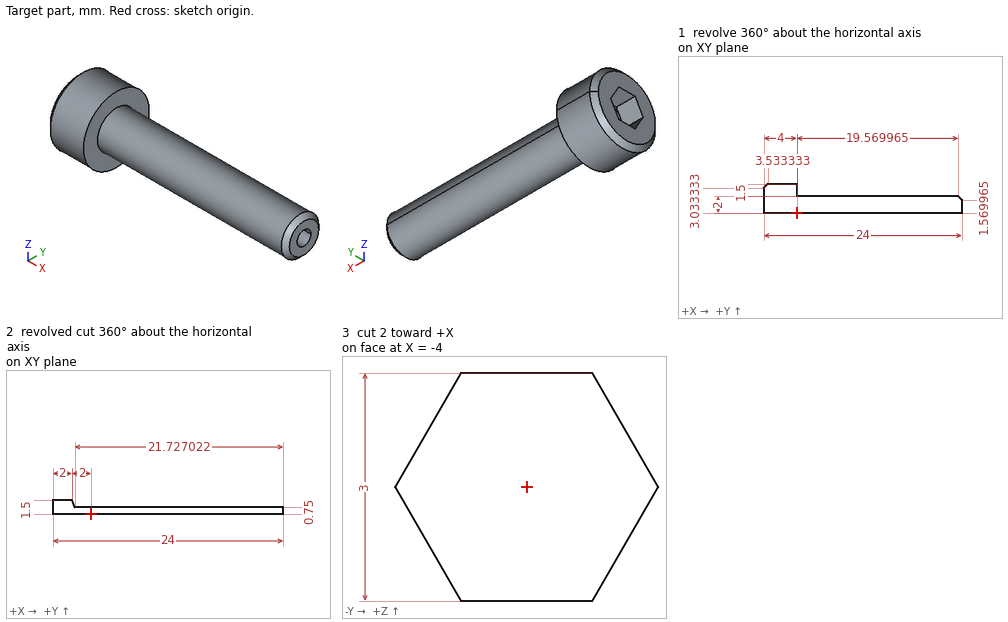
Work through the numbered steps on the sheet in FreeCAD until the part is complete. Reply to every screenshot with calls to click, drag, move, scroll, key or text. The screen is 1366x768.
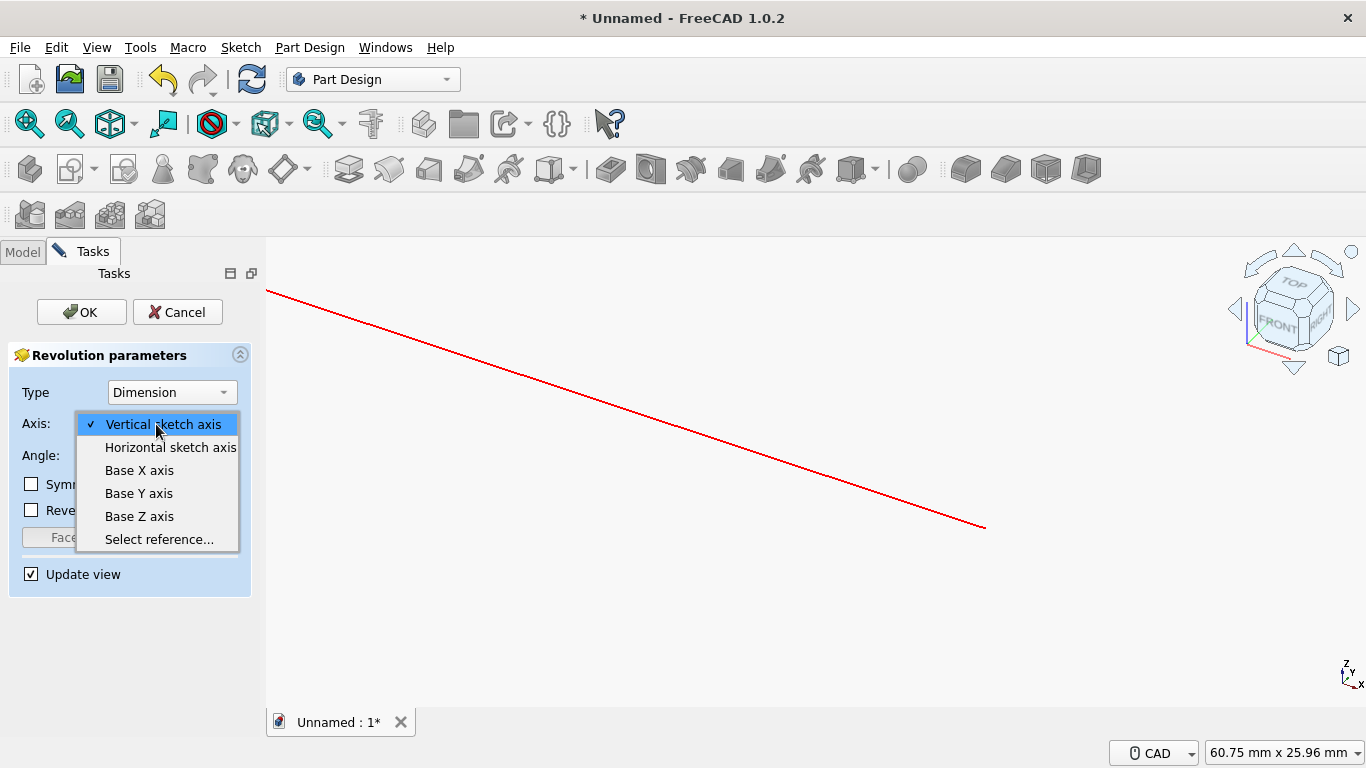
click(156, 448)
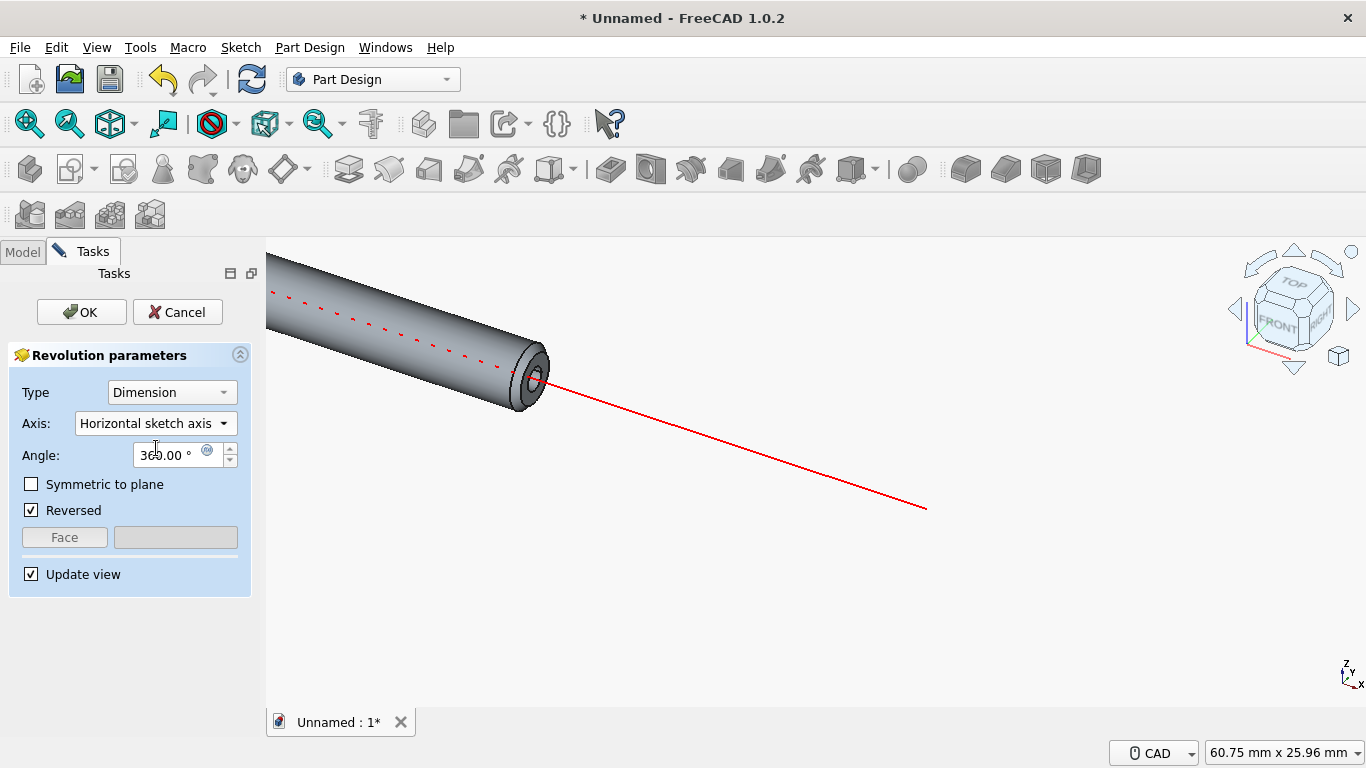
click(82, 312)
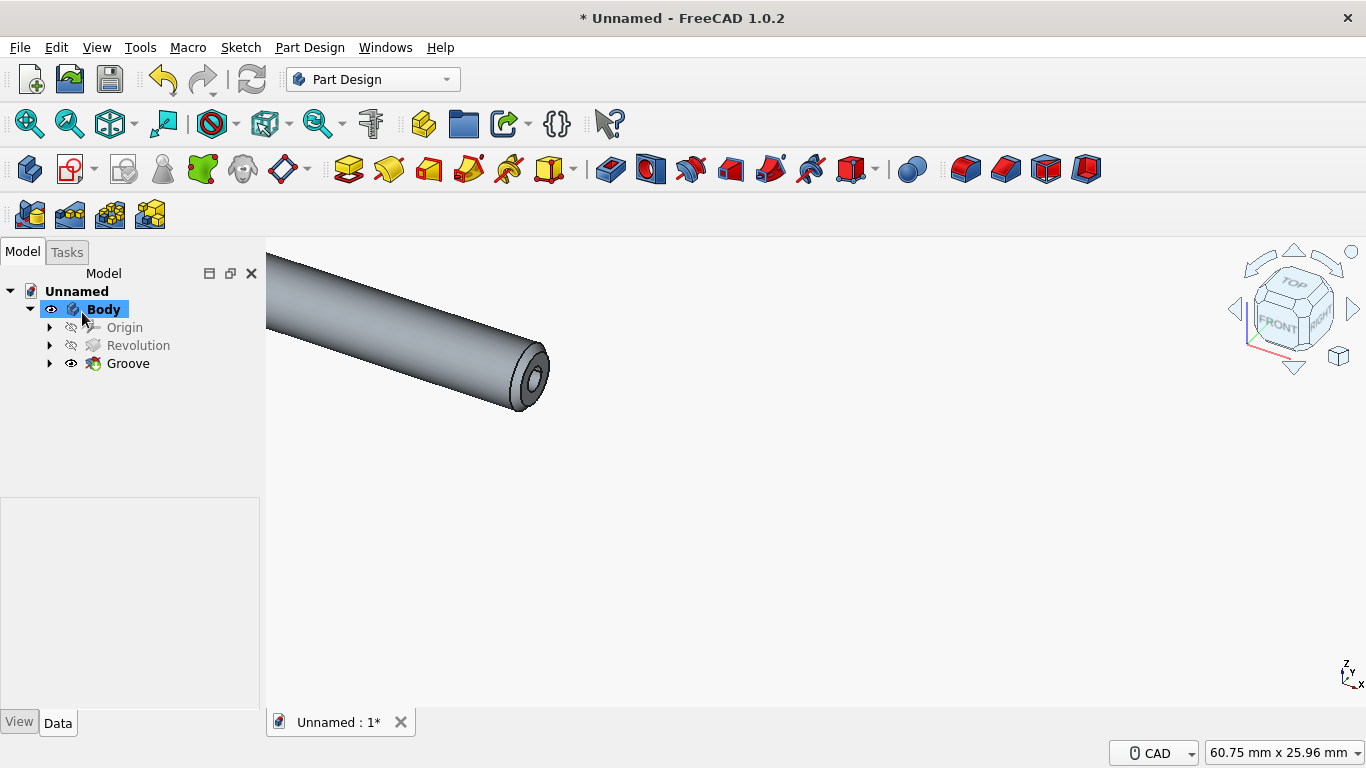
click(30, 124)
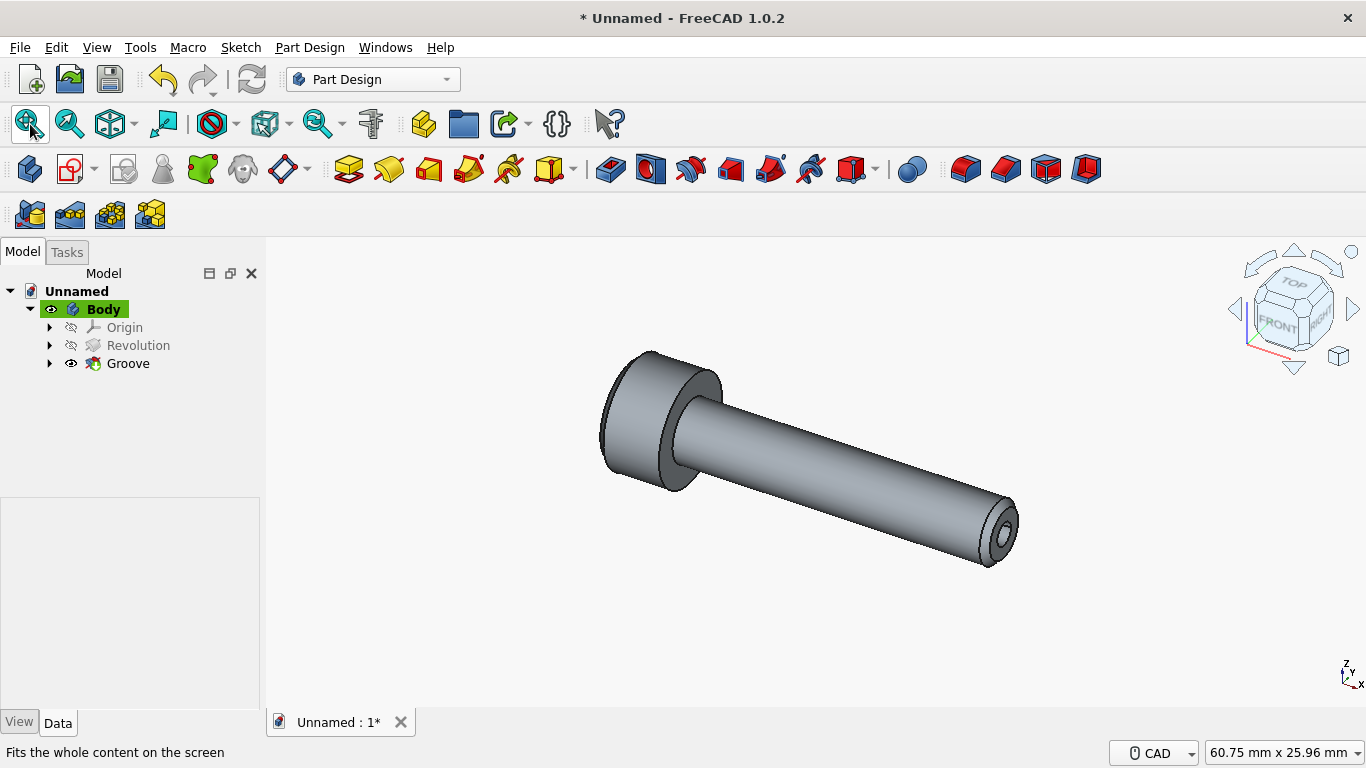
key(6)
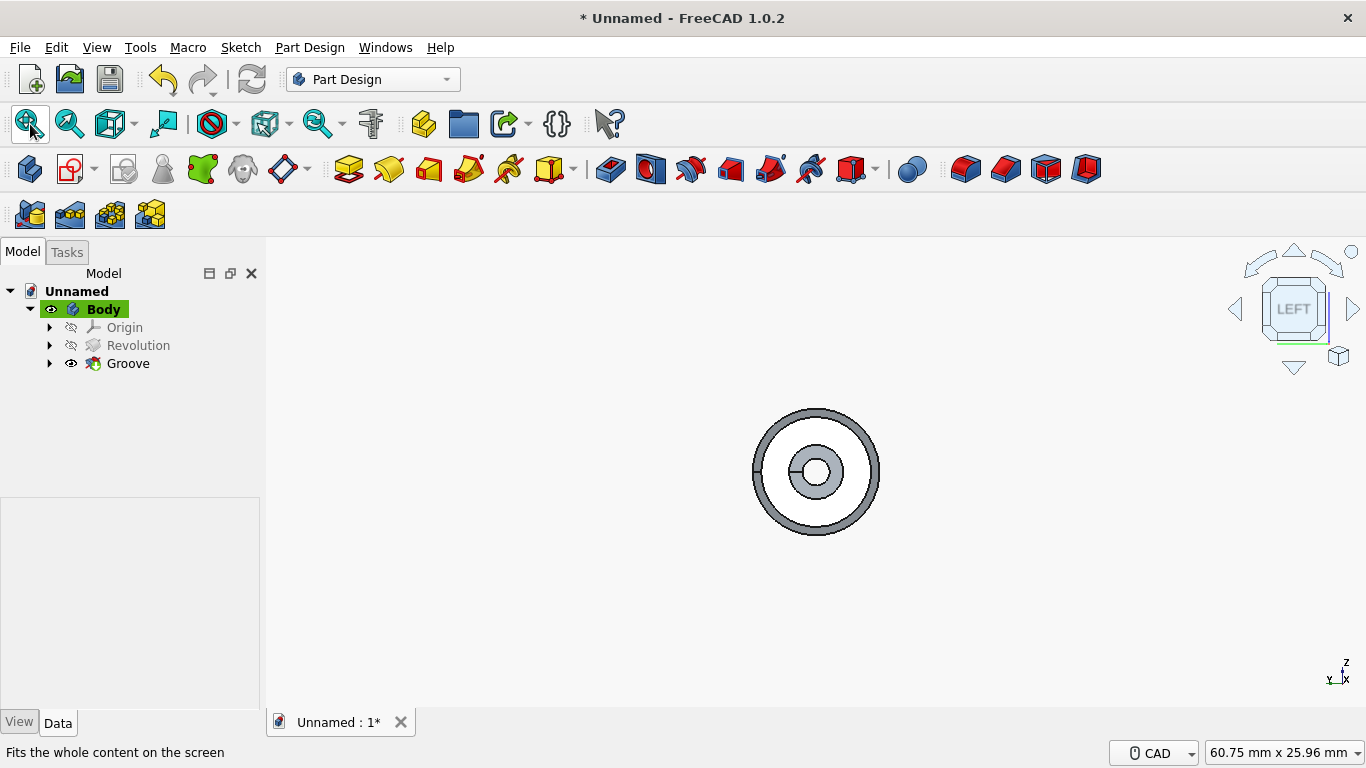
click(30, 124)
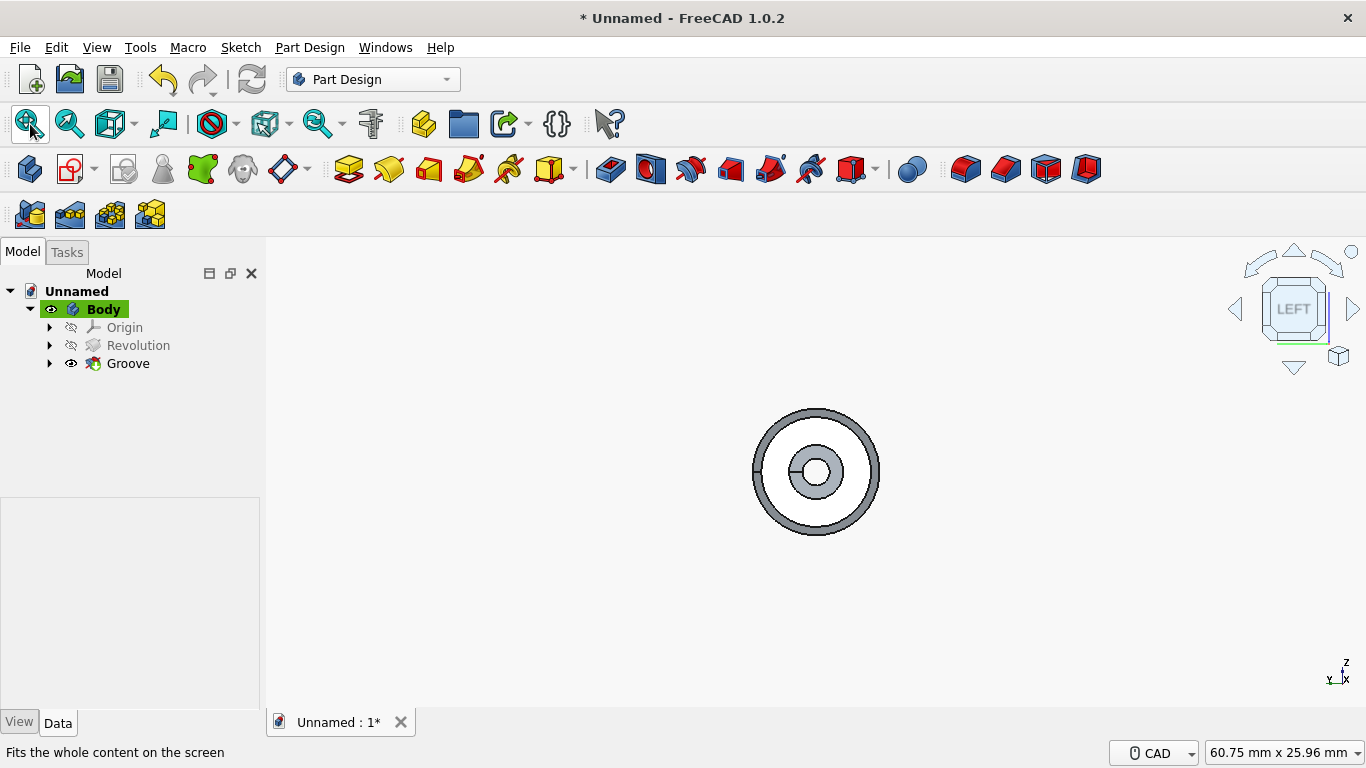
click(785, 440)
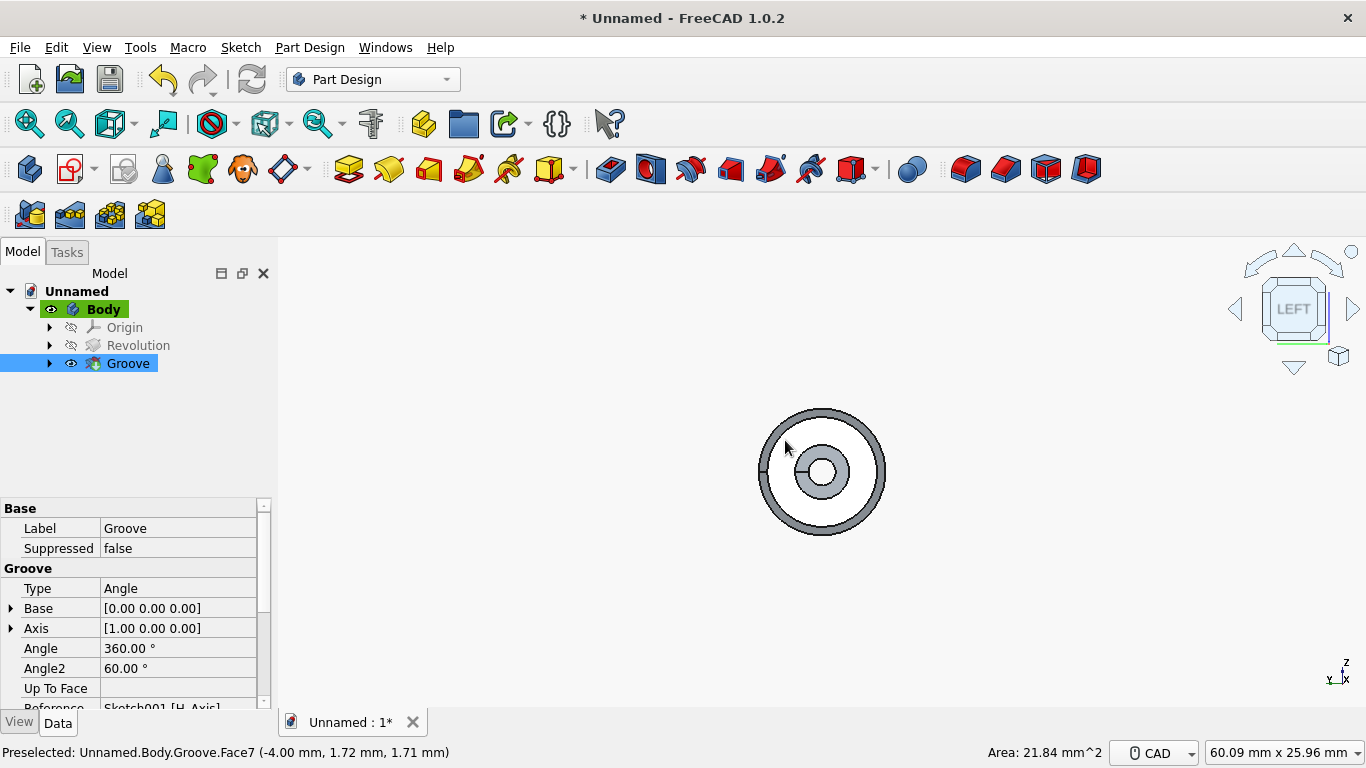
click(70, 170)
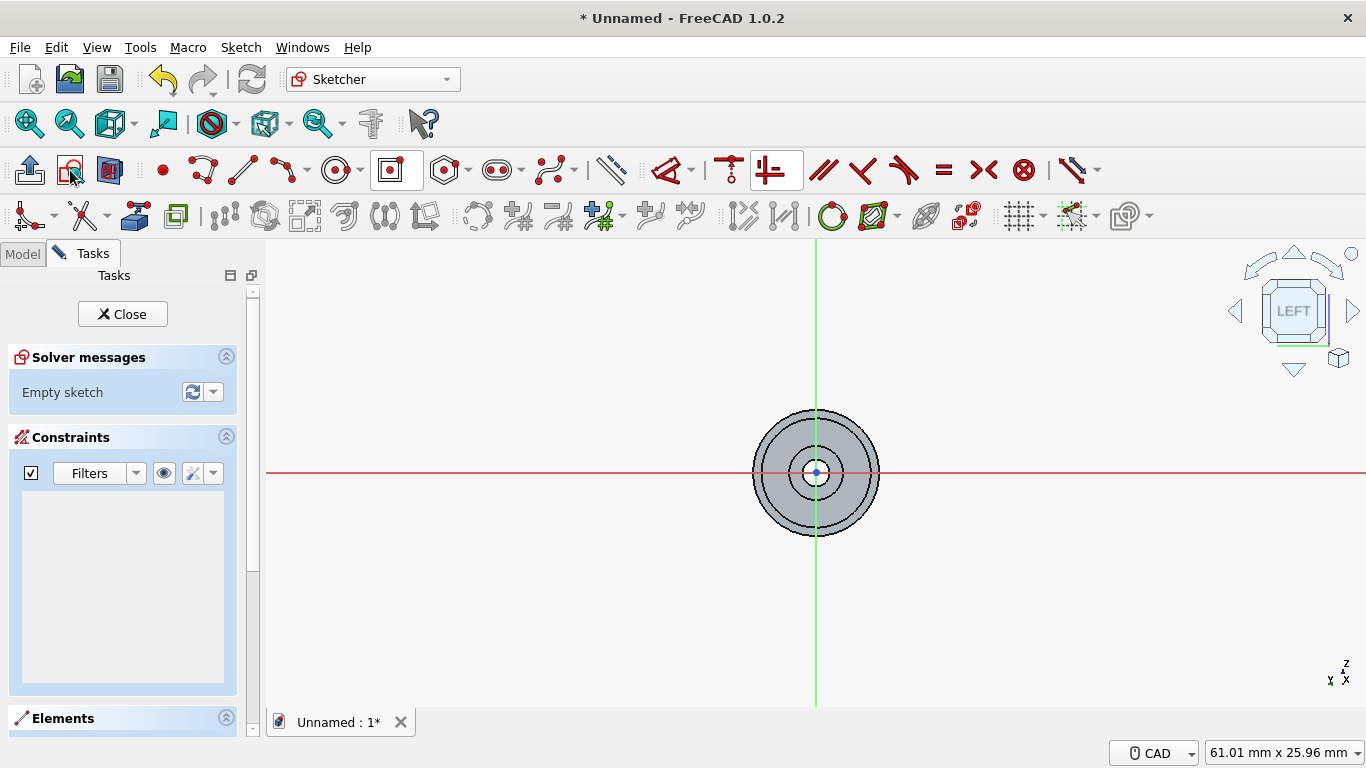
scroll(833, 473, up, 8)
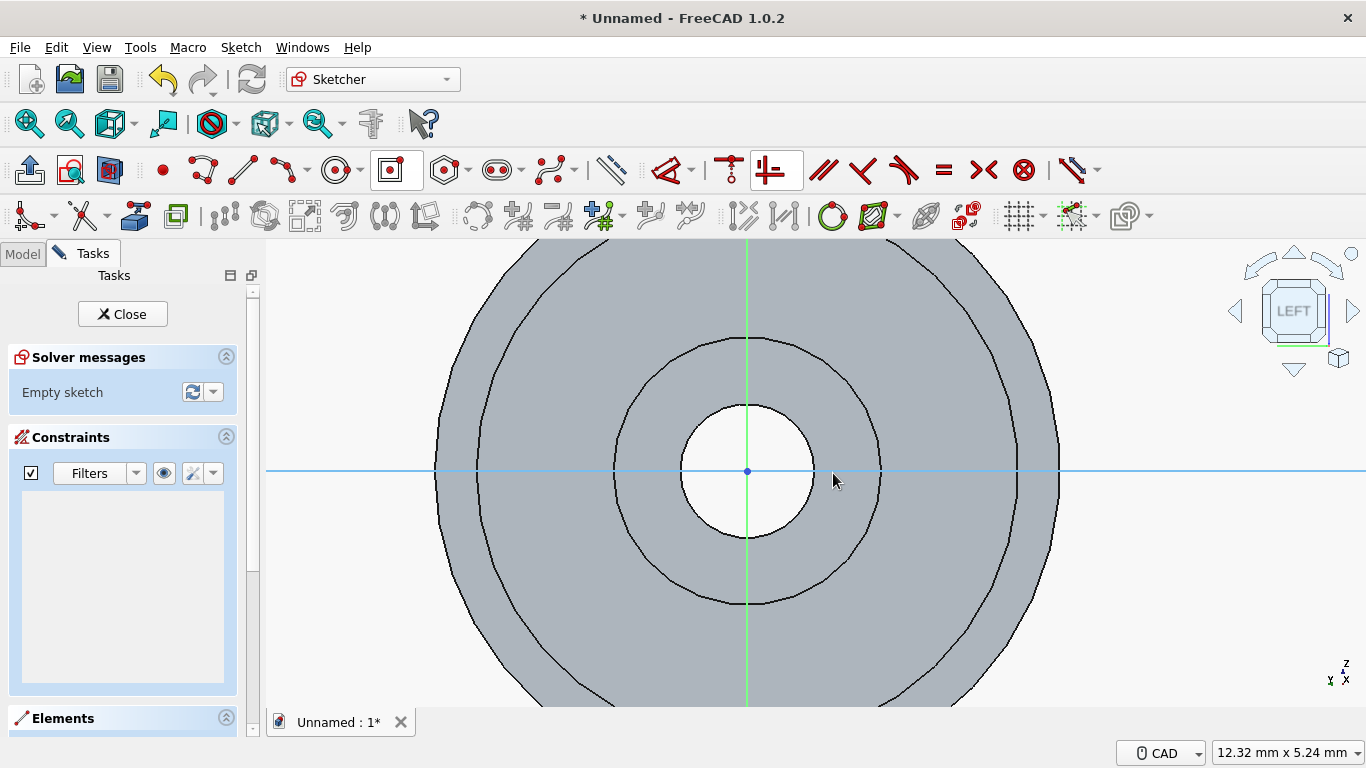
click(444, 170)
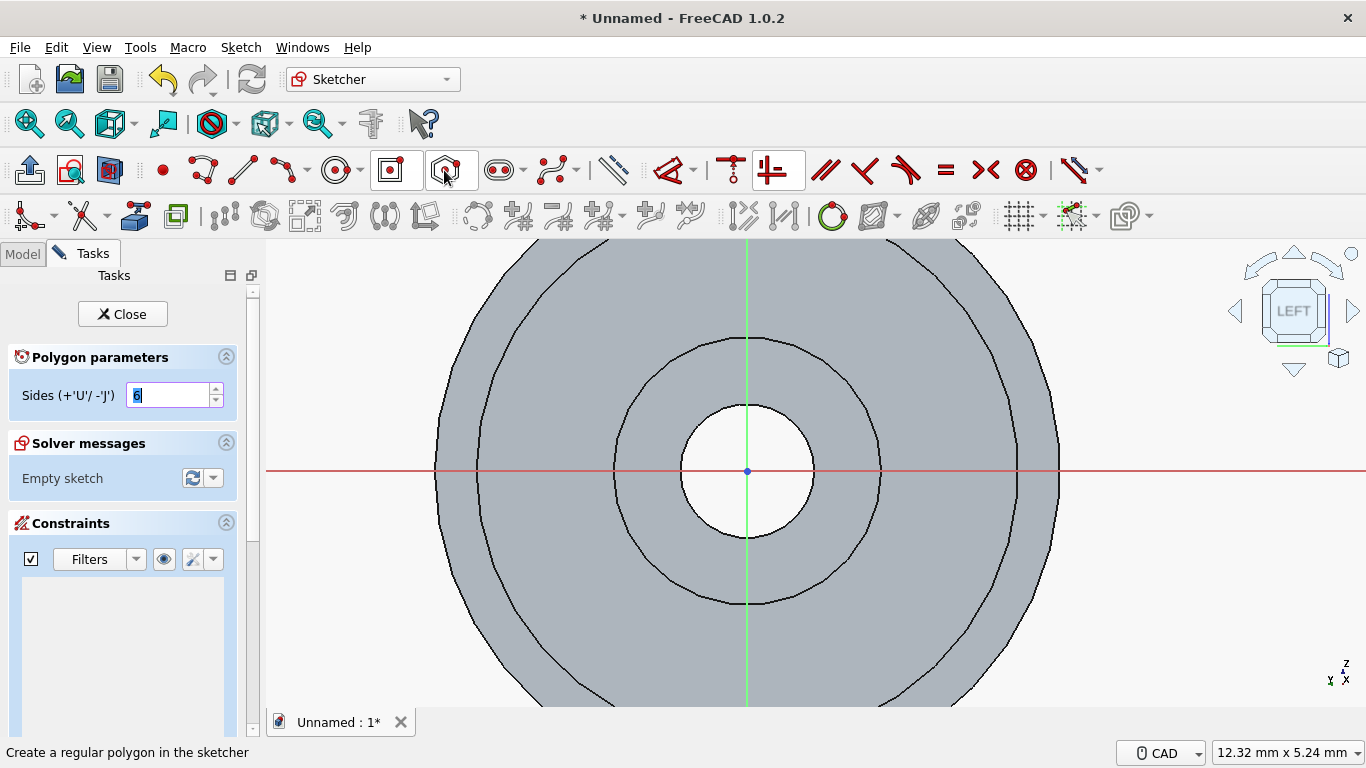
click(747, 471)